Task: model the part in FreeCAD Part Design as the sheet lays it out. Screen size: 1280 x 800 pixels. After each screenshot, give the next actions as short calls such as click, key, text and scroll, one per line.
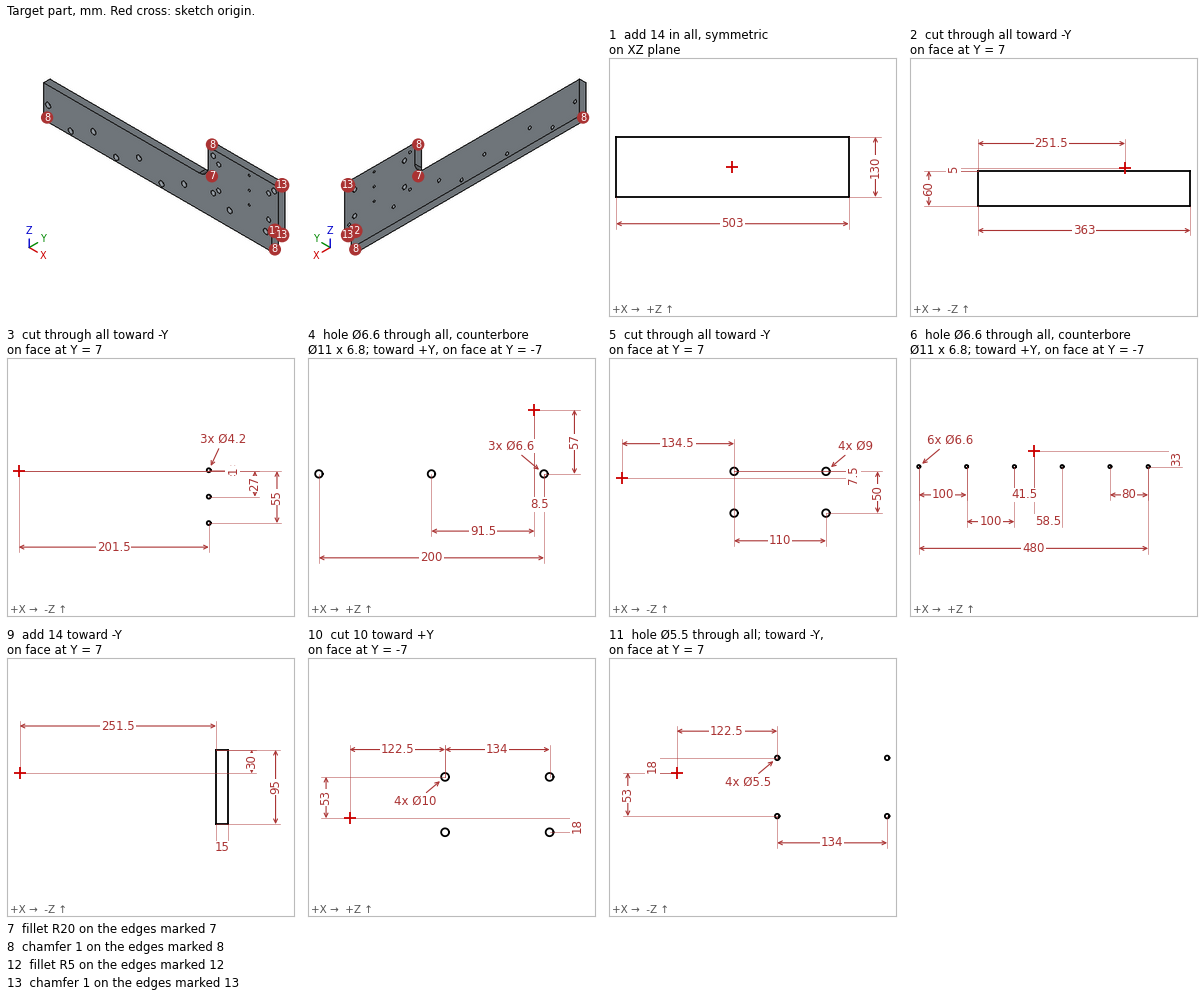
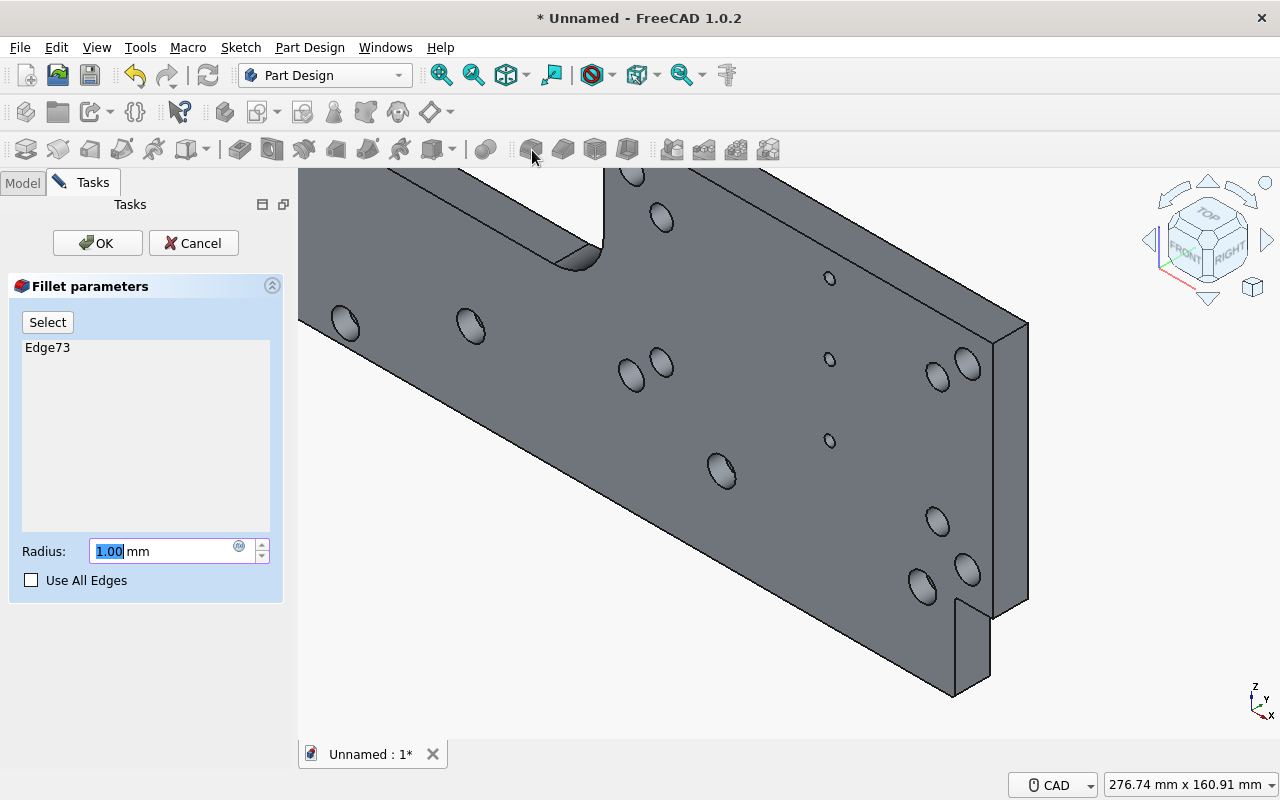
text(5)
key(Tab)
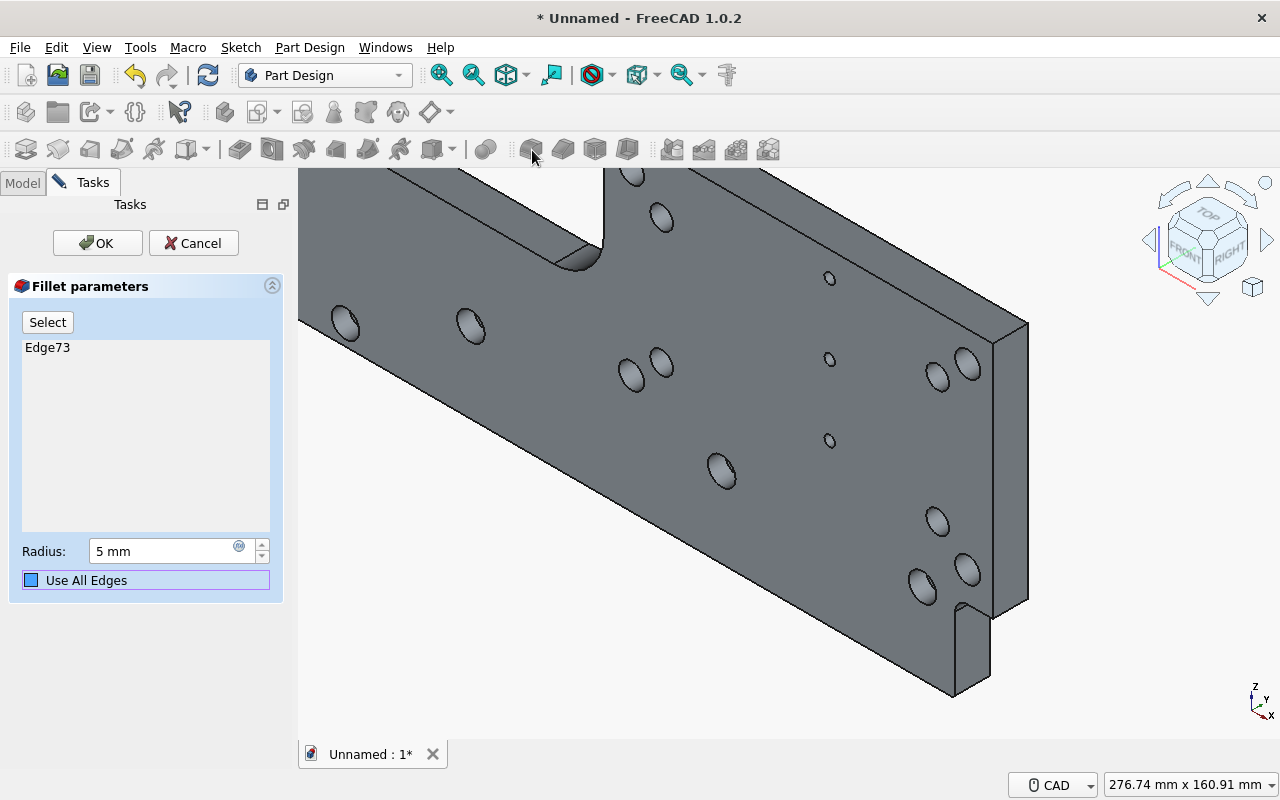
click(98, 243)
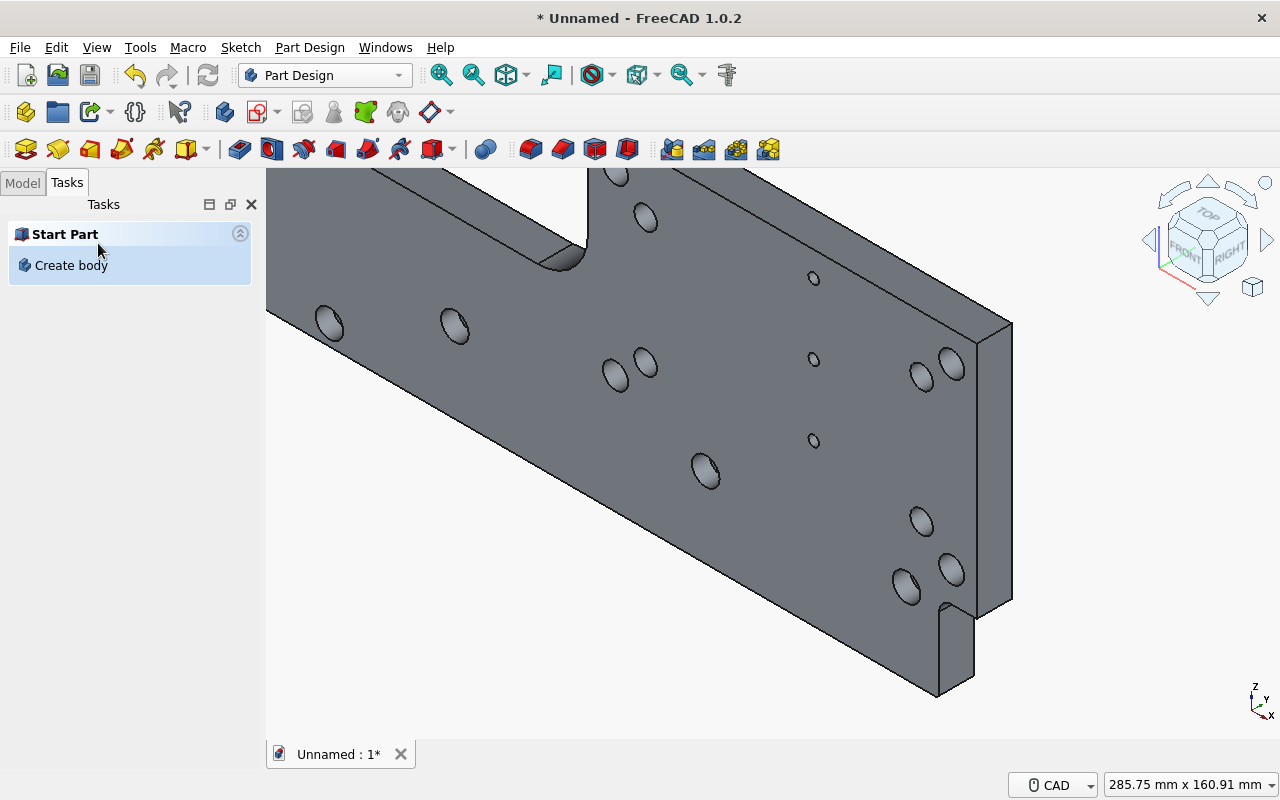
click(442, 76)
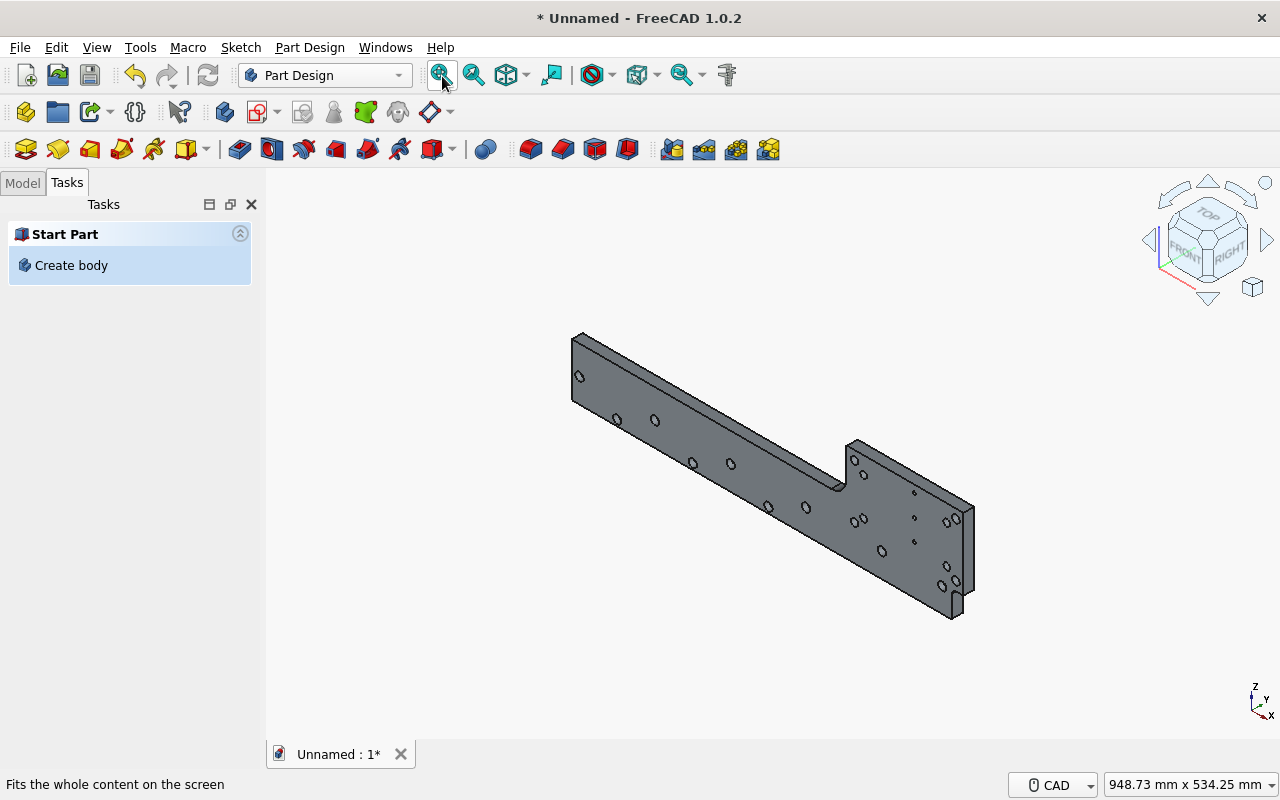
click(970, 508)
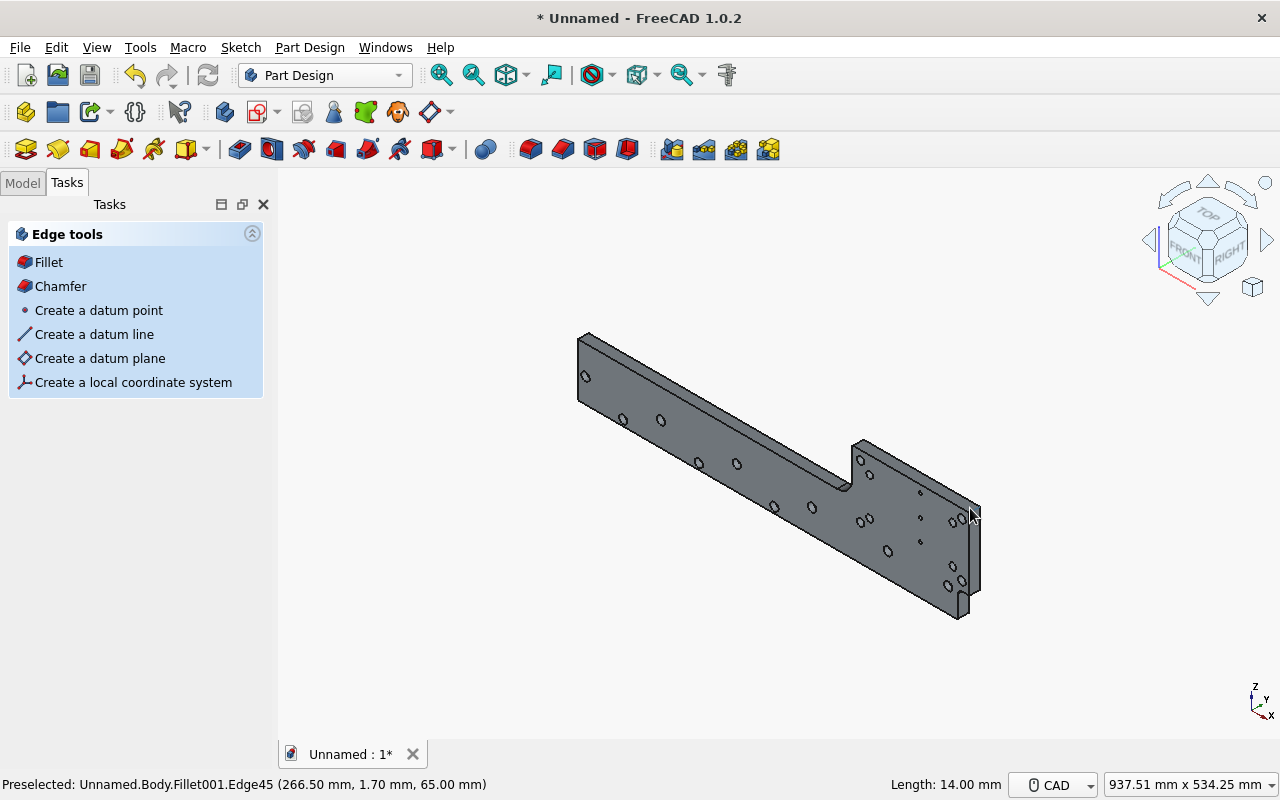
scroll(975, 592, up, 5)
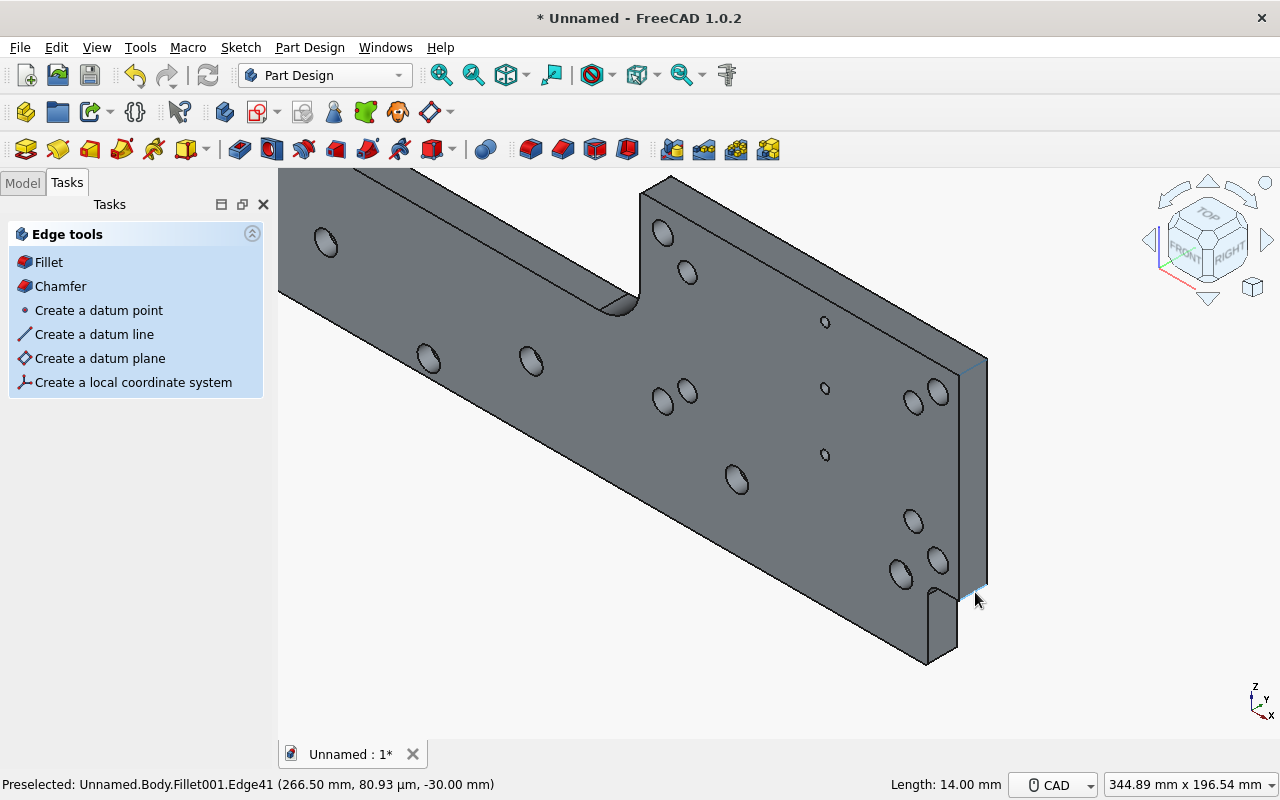
key(v)
key(f)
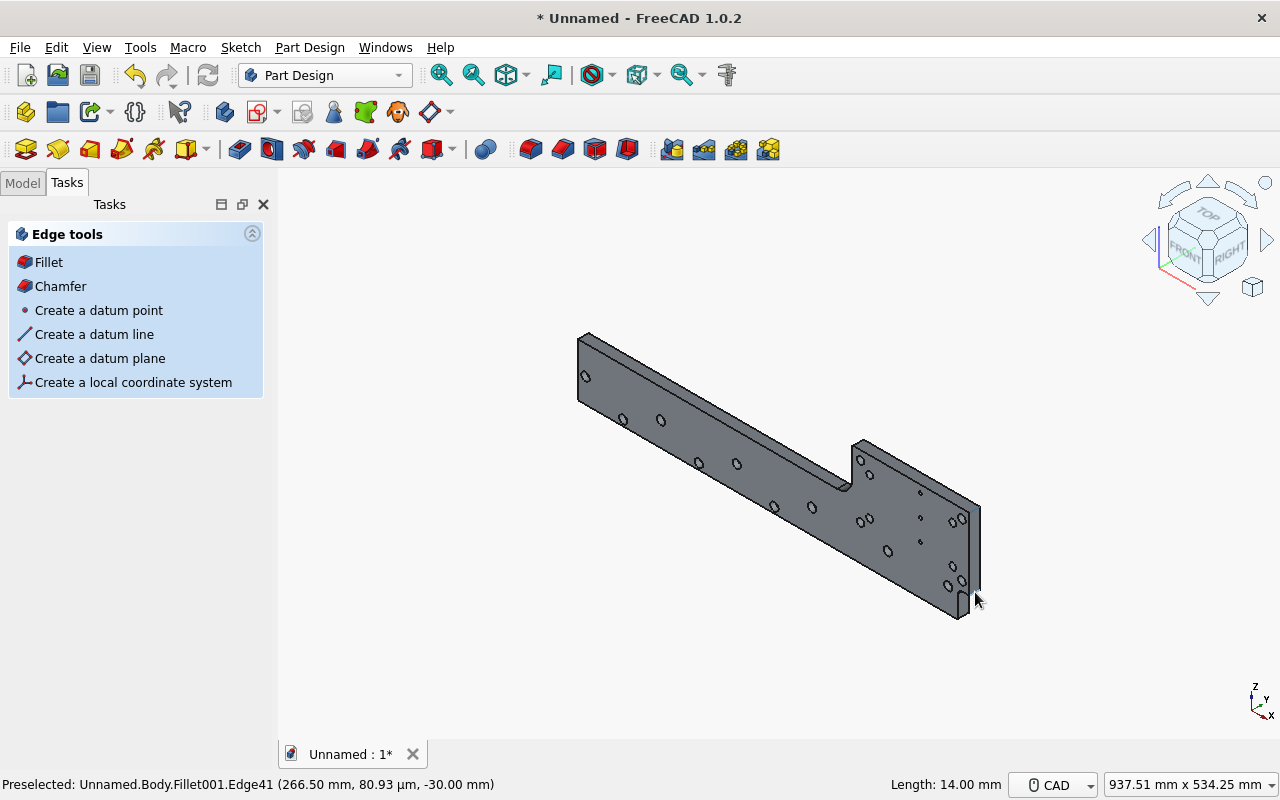
key(2)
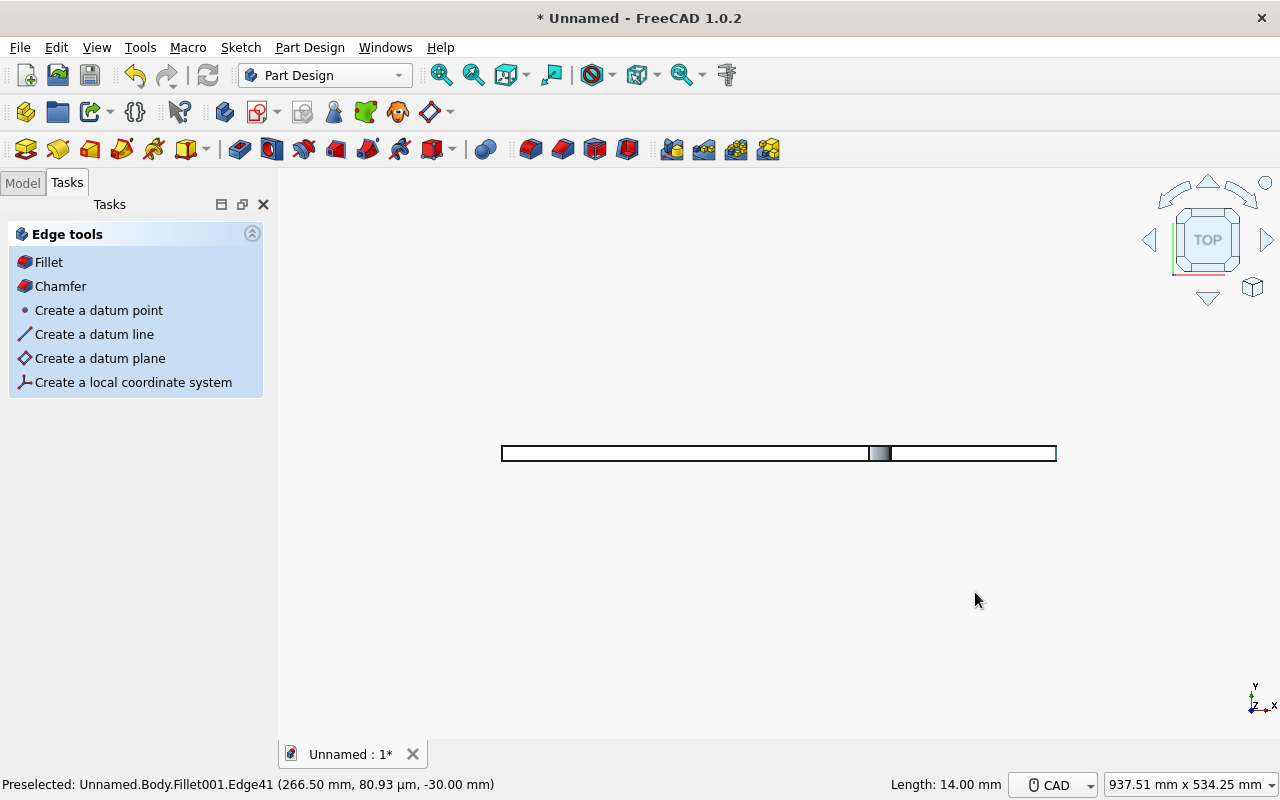
scroll(1056, 452, up, 5)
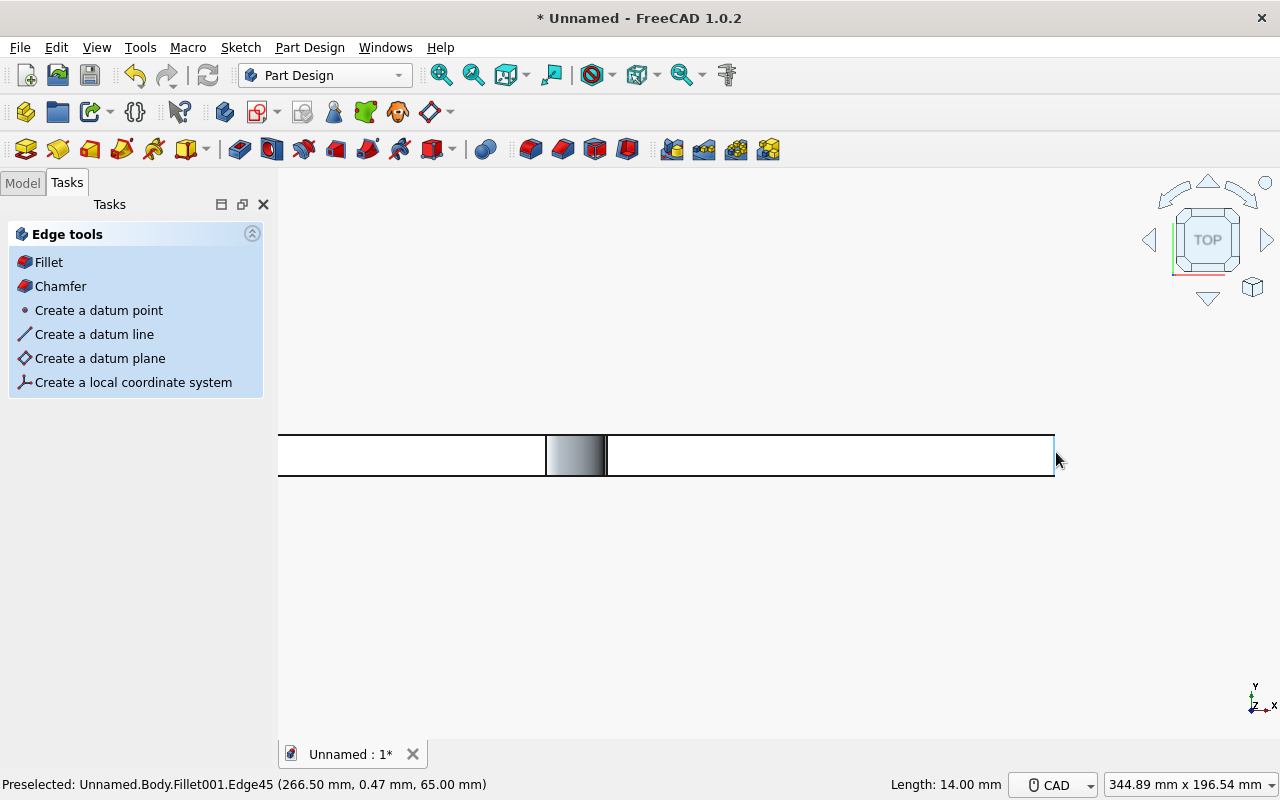
key(v)
key(f)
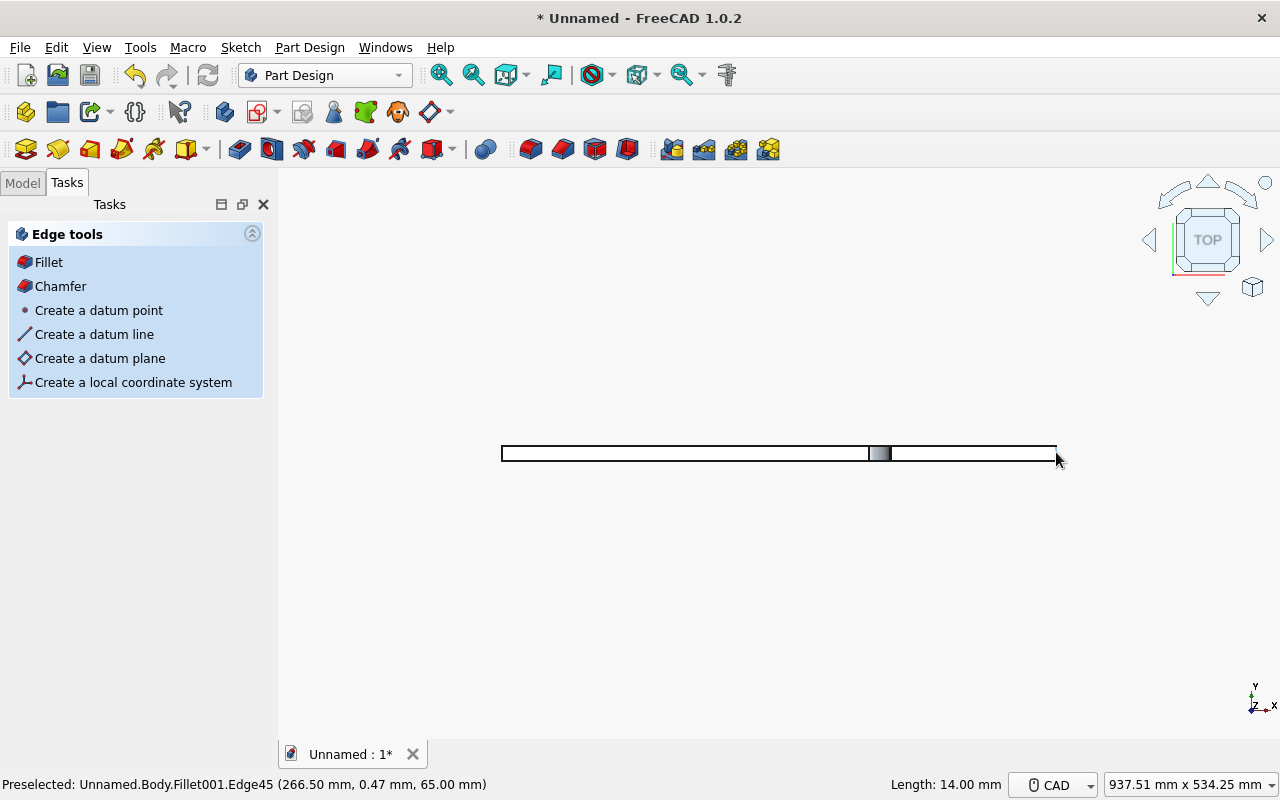
key(0)